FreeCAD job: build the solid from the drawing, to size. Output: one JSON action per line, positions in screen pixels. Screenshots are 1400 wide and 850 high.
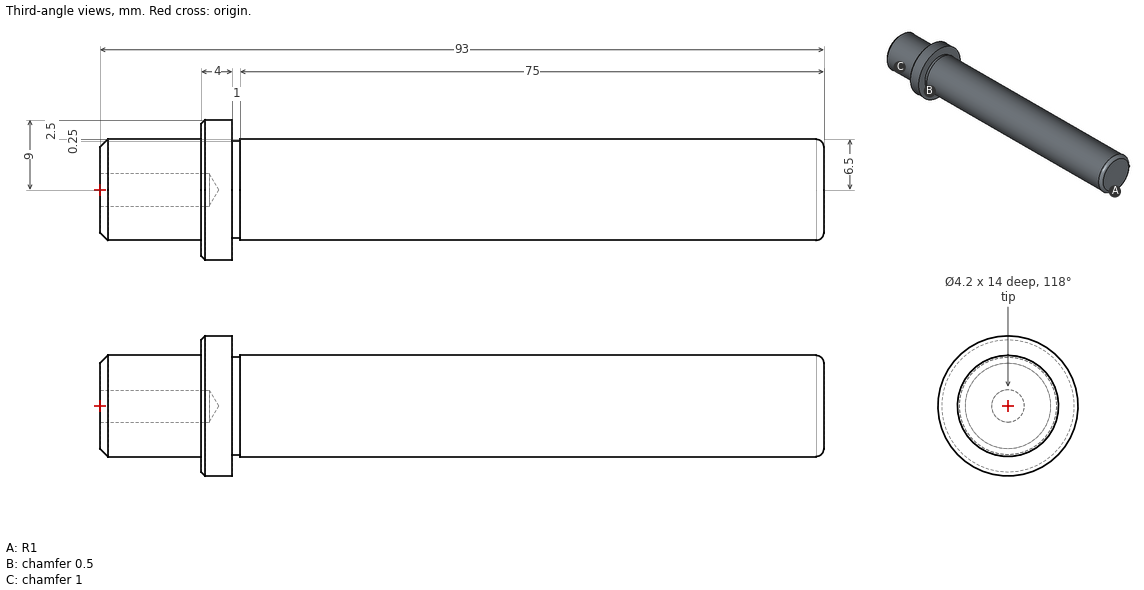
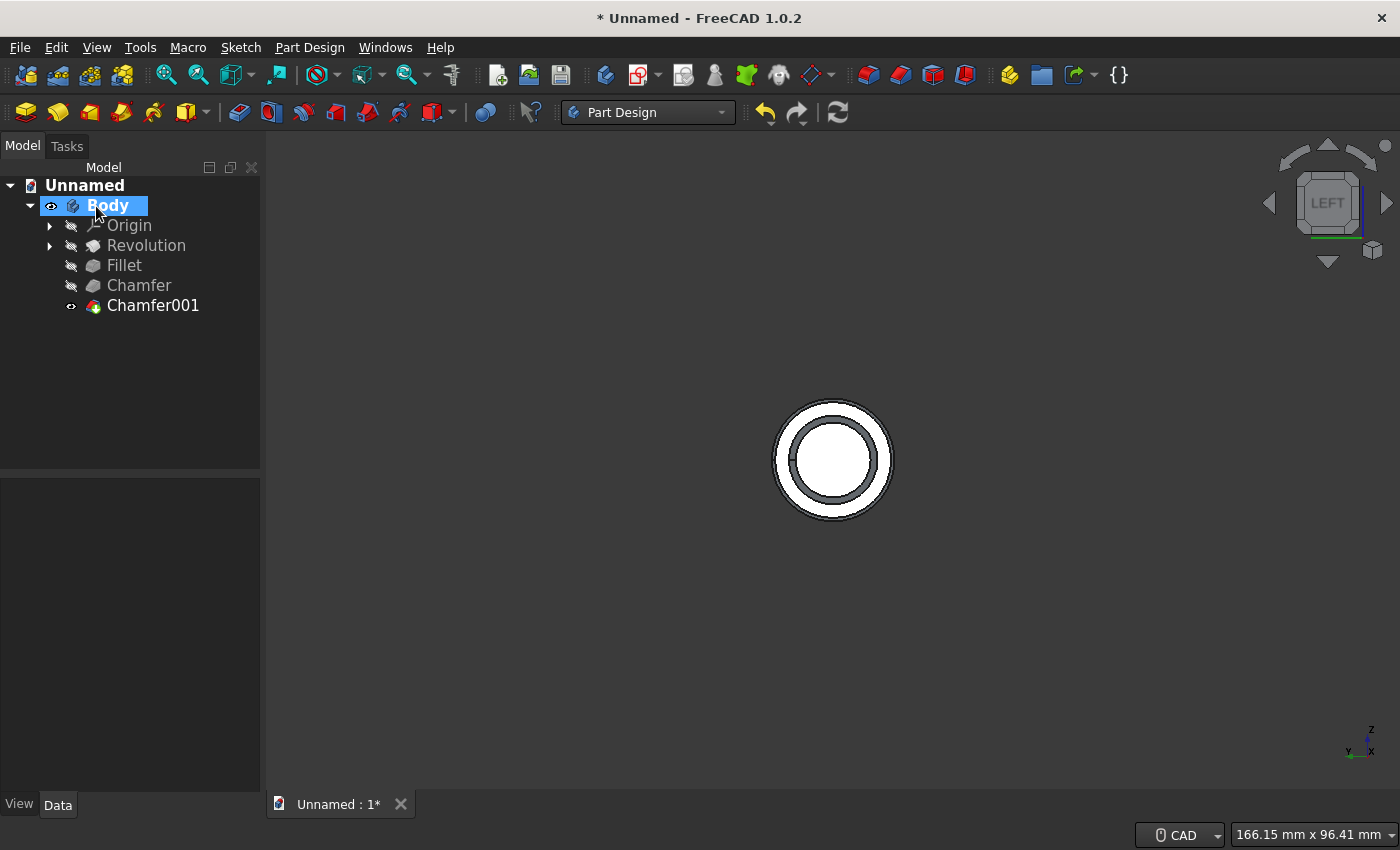
{"action": "left_click", "coordinate": [833, 459]}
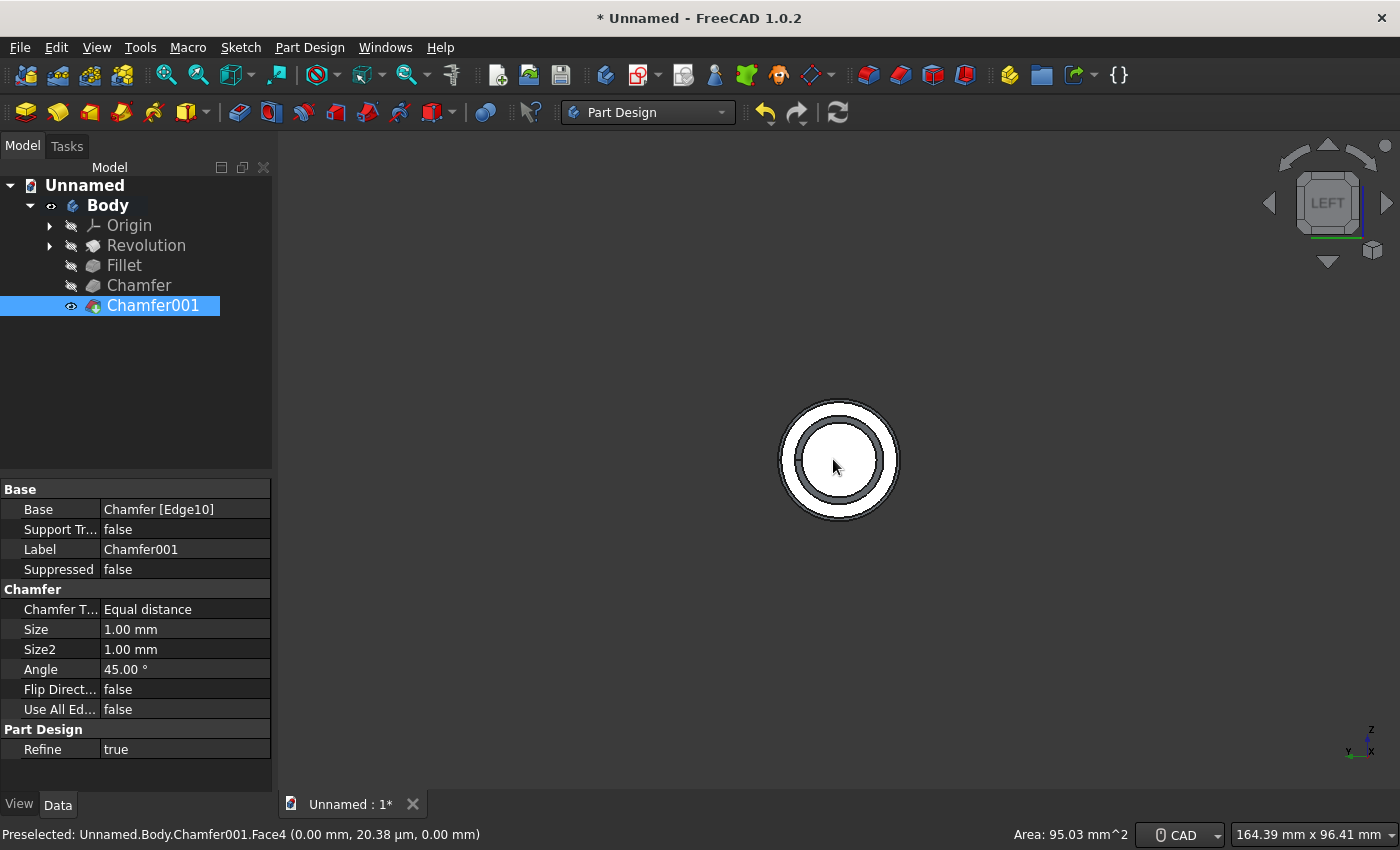
{"action": "left_click", "coordinate": [638, 76]}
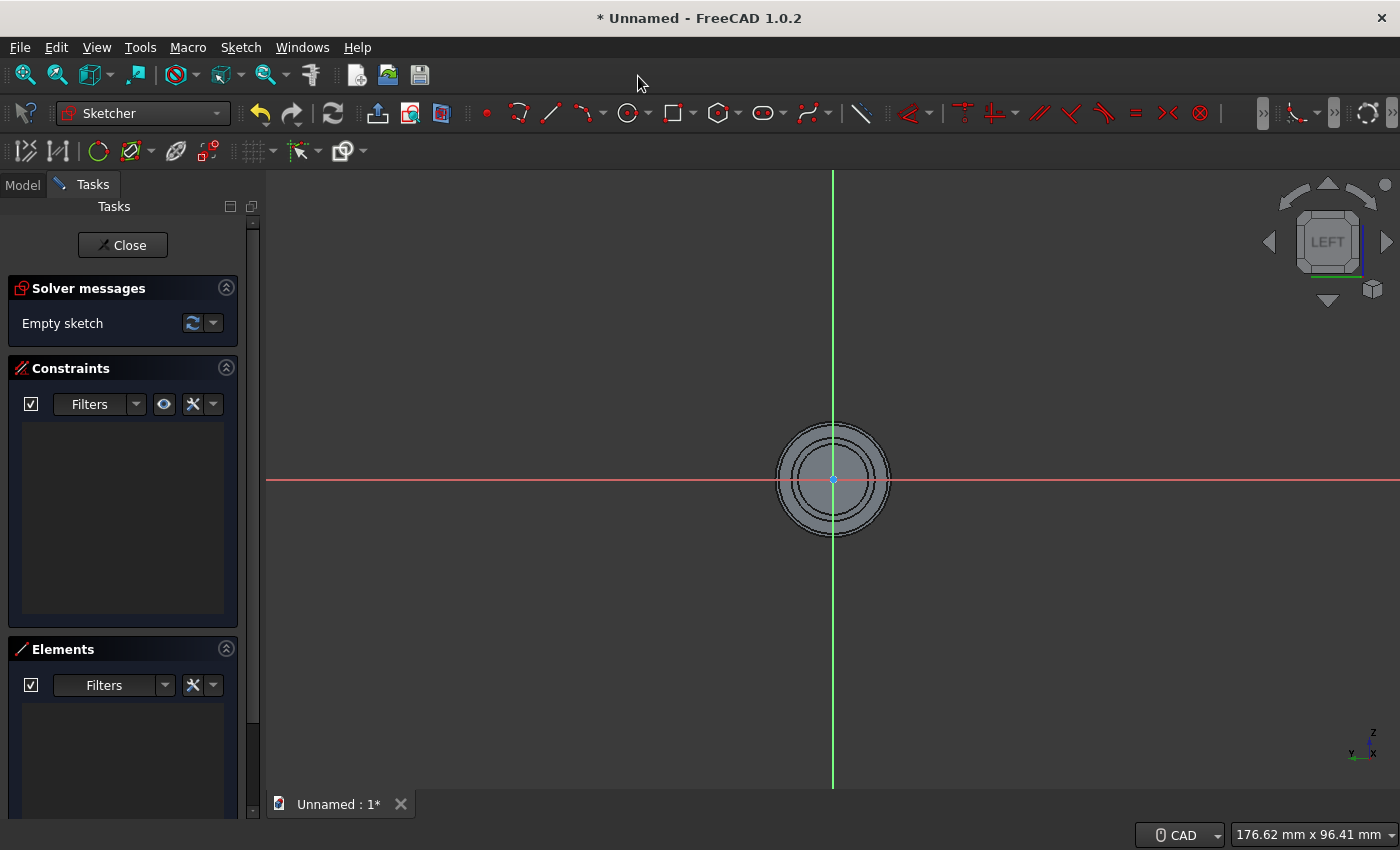
{"action": "scroll", "coordinate": [839, 480], "scroll_direction": "up", "scroll_amount": 13}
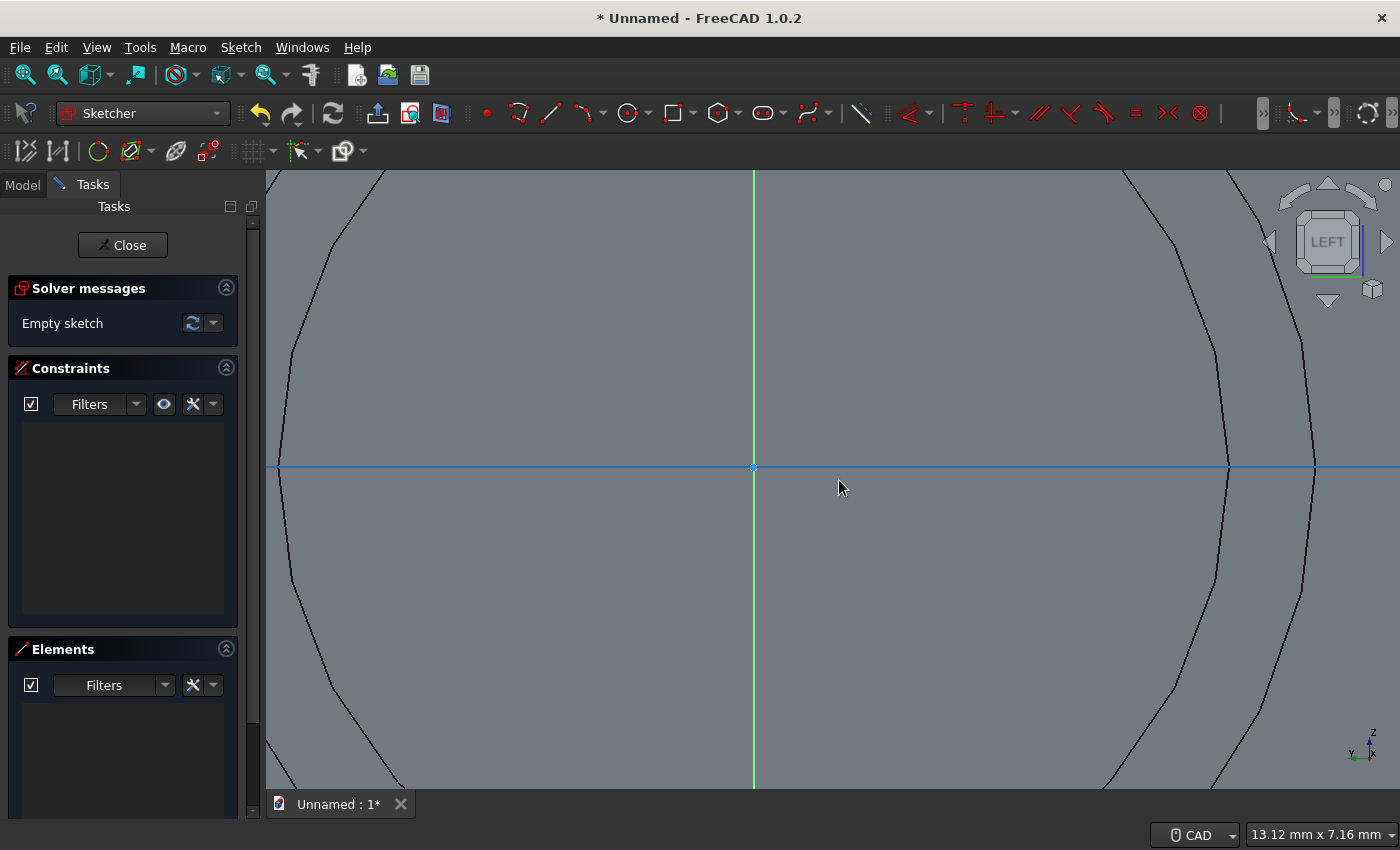
{"action": "key", "text": "g c"}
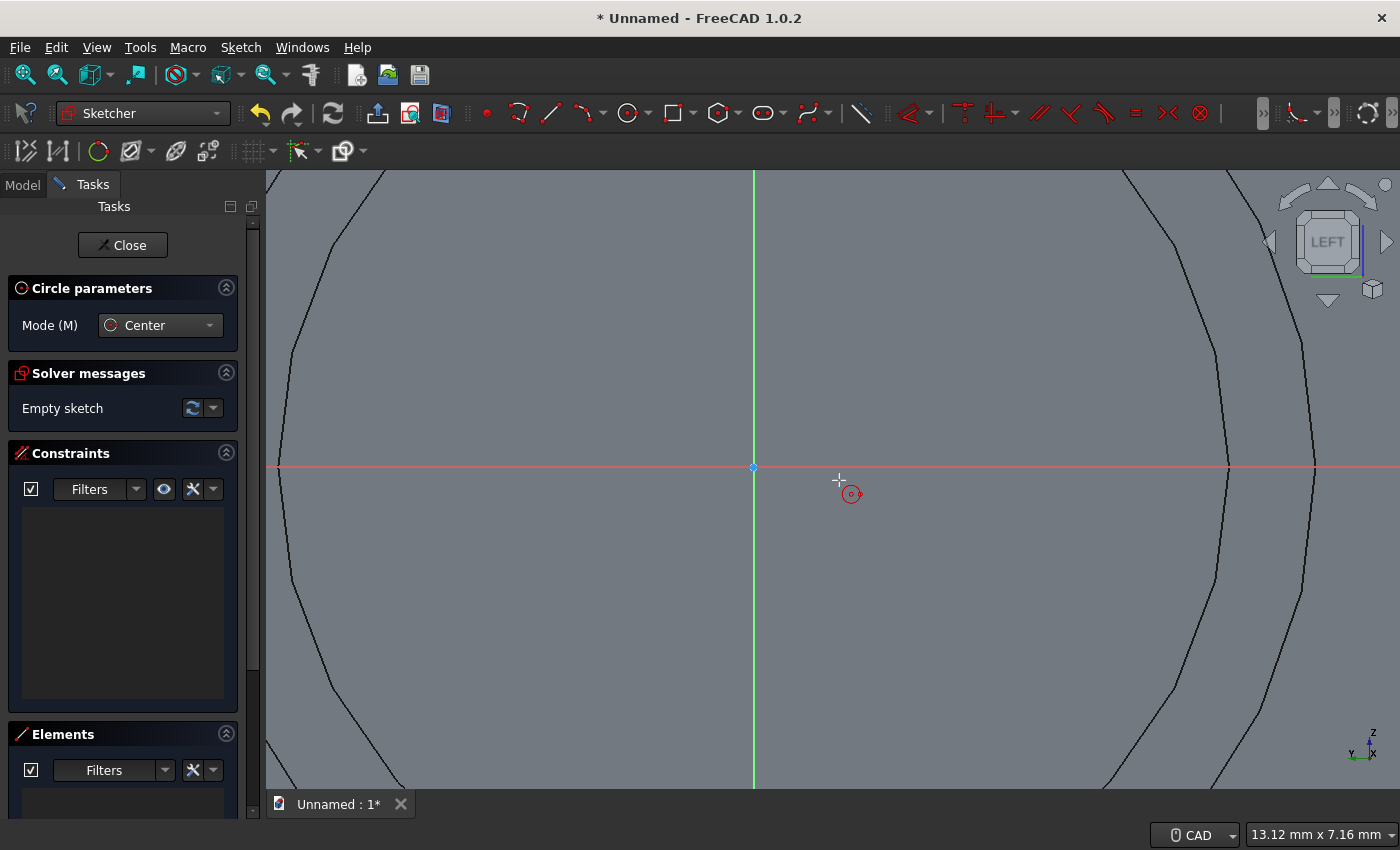
{"action": "left_click", "coordinate": [754, 467]}
{"action": "mouse_move", "coordinate": [882, 339]}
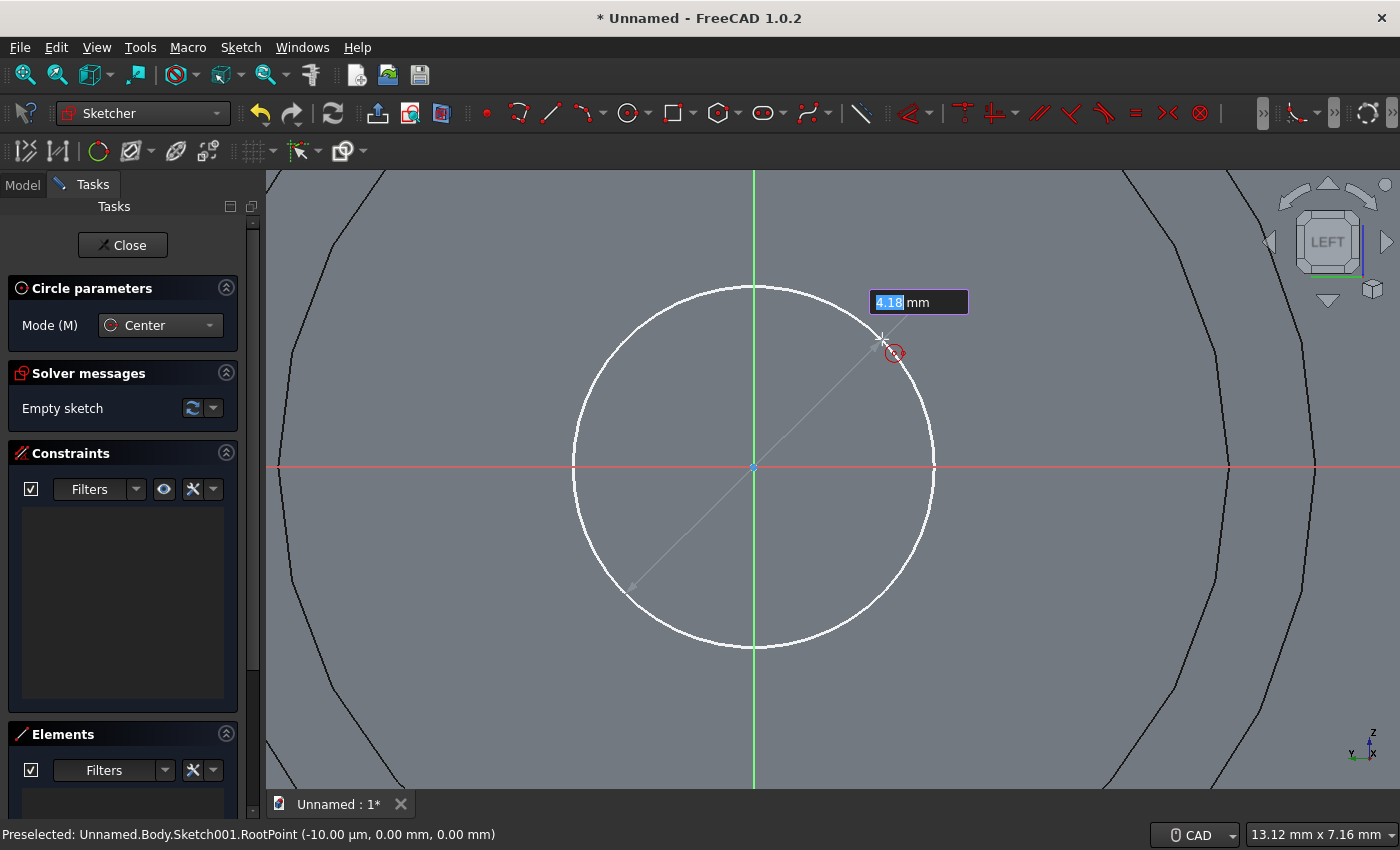
{"action": "type", "text": "4.2"}
{"action": "key", "text": "Return"}
{"action": "key", "text": "Escape"}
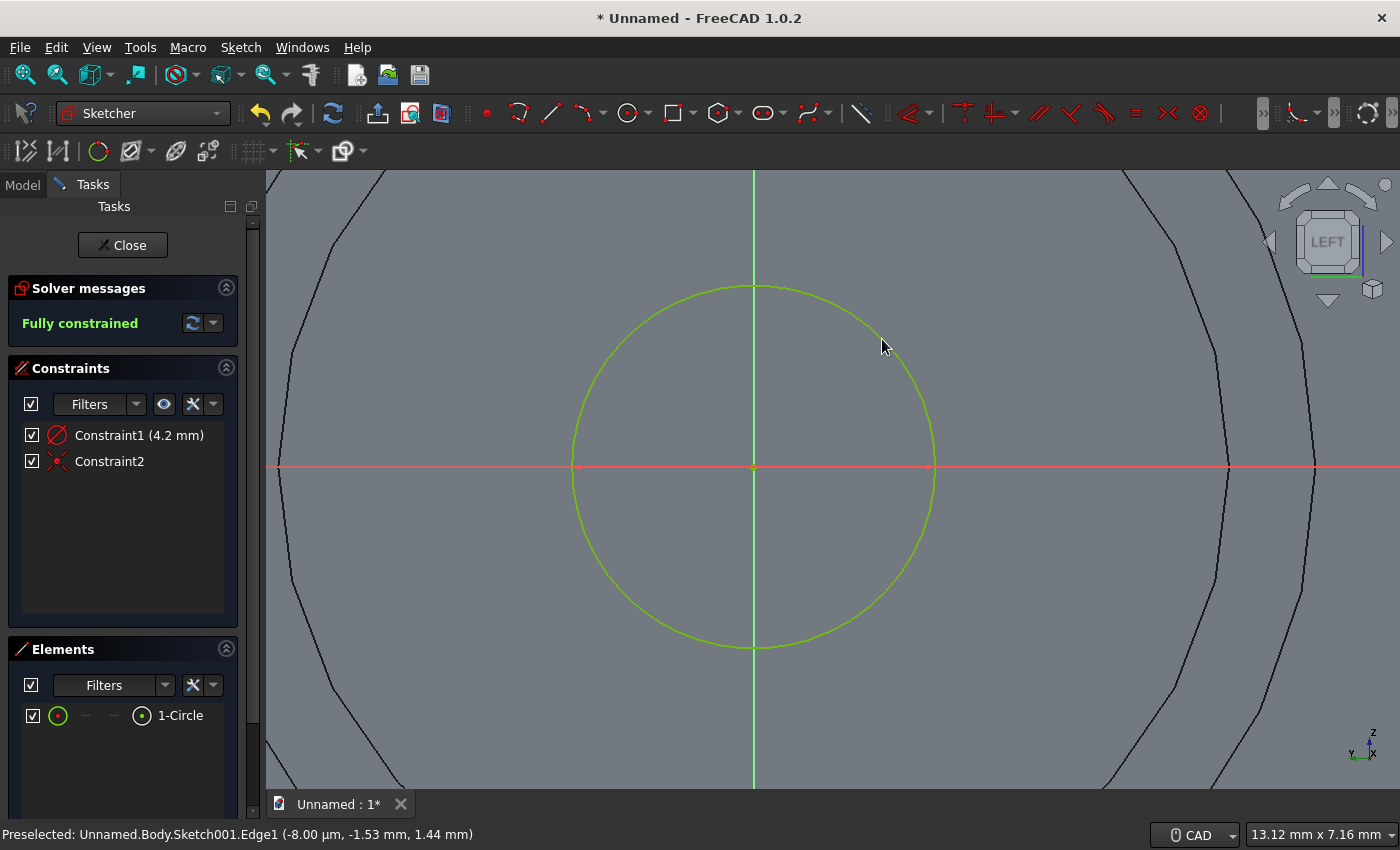
{"action": "left_click", "coordinate": [123, 245]}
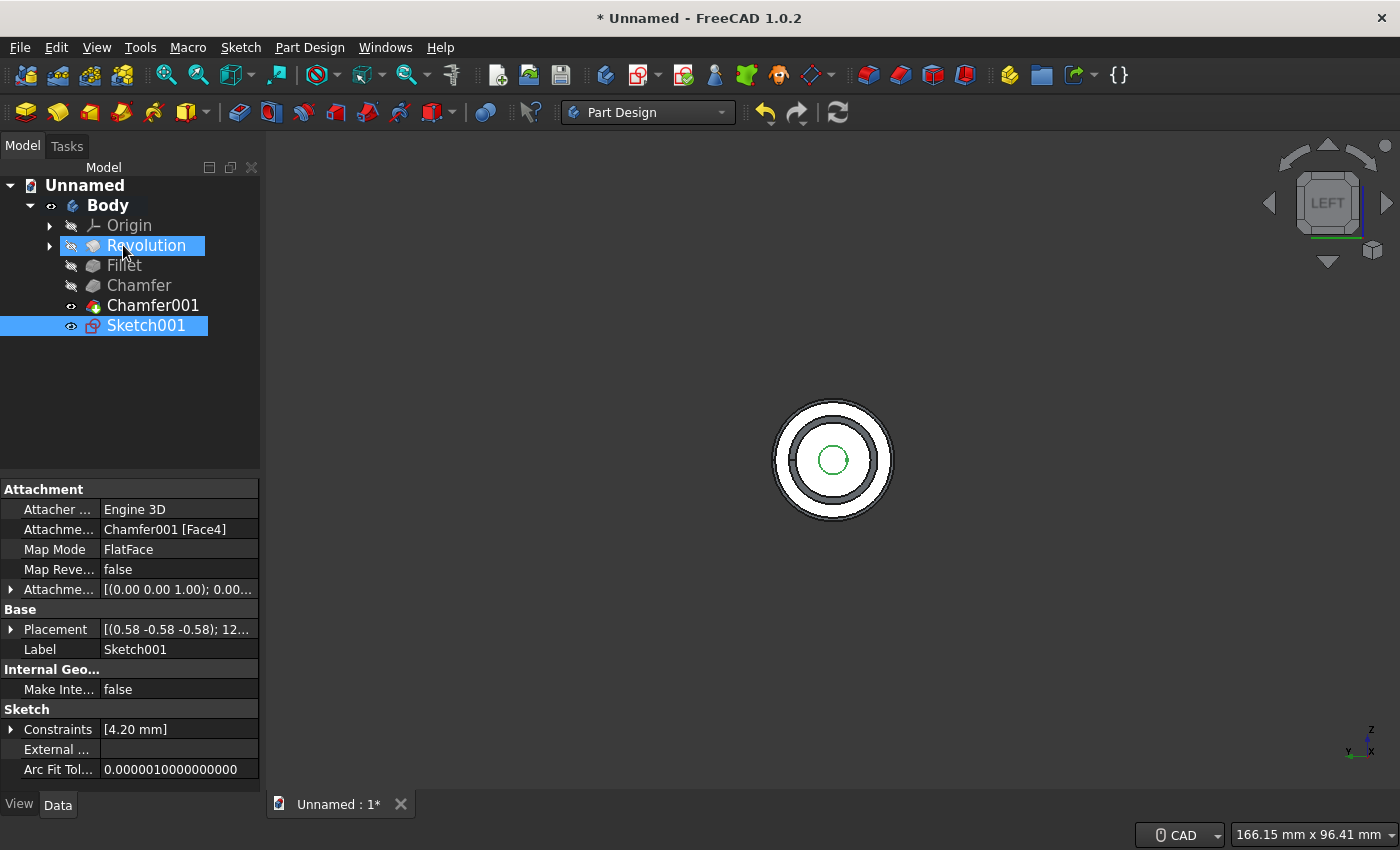
{"action": "left_click", "coordinate": [272, 112]}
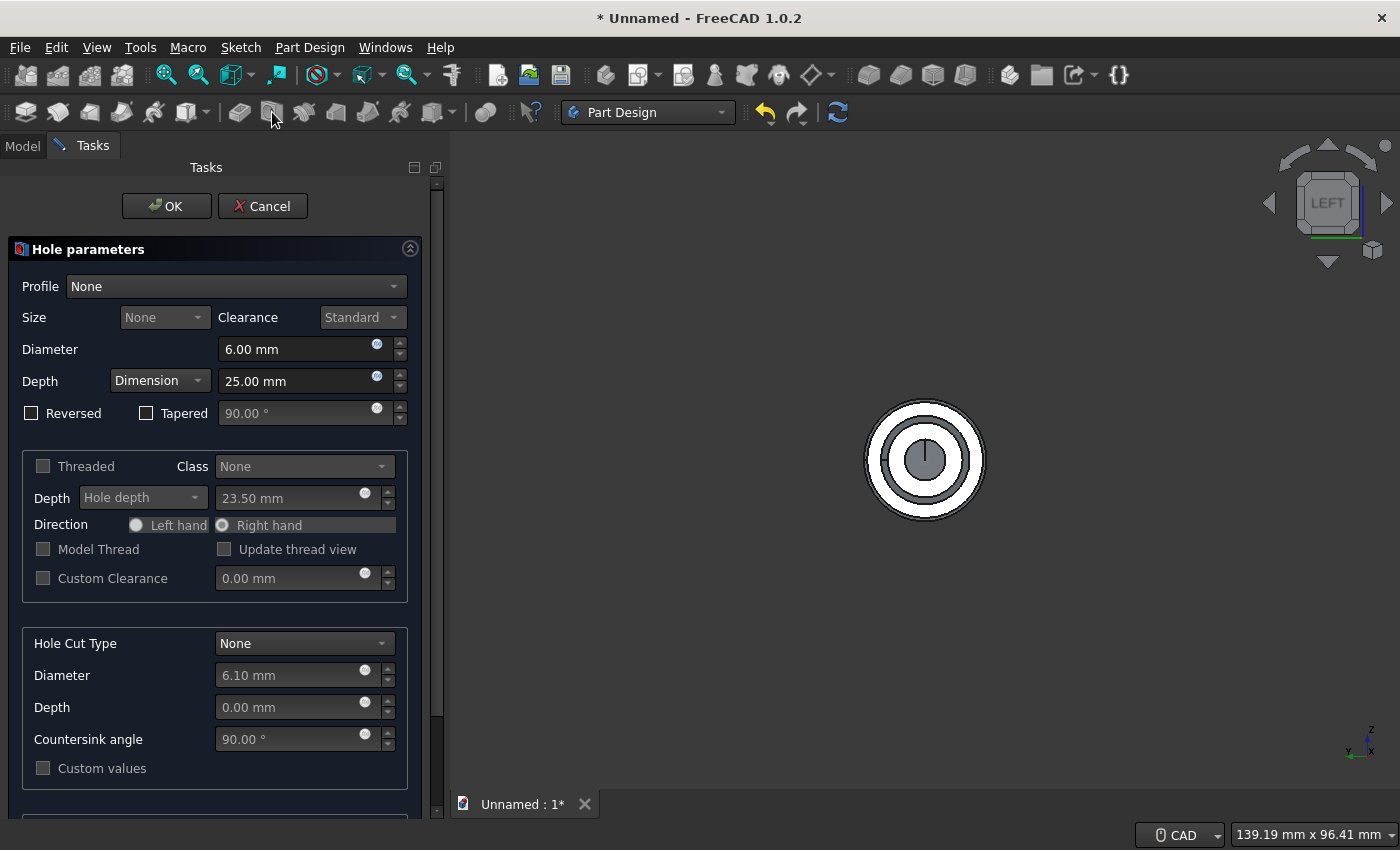
{"action": "triple_click", "coordinate": [305, 349]}